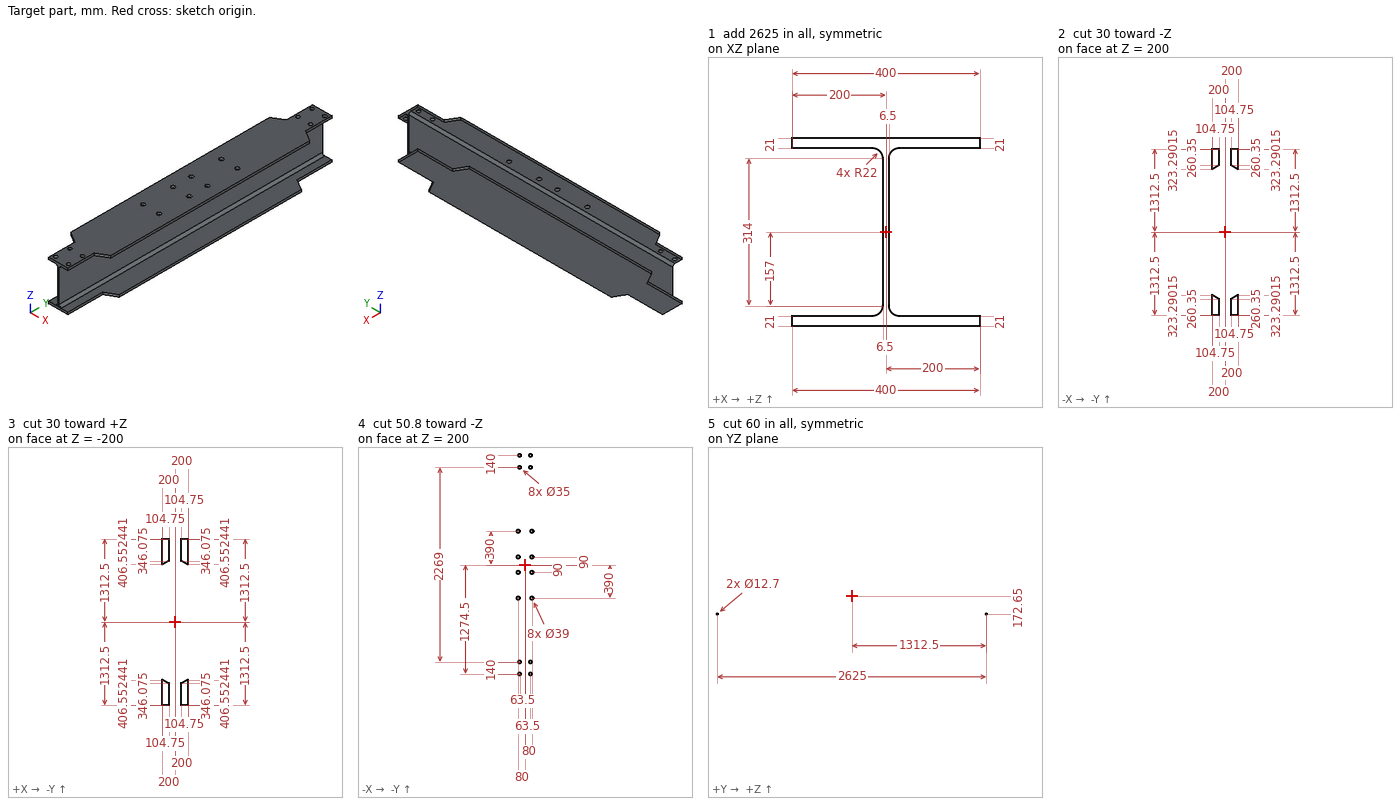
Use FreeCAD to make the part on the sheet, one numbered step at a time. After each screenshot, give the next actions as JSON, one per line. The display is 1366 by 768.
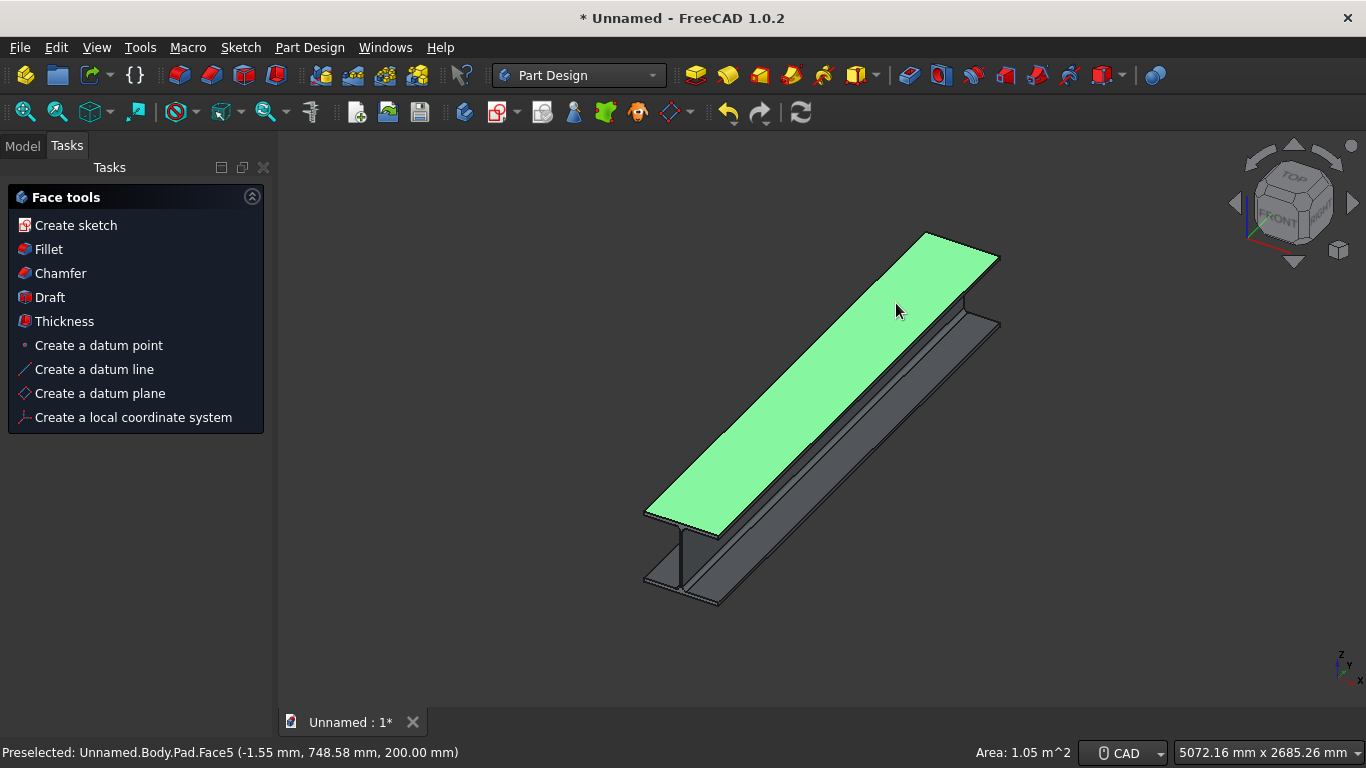
{"action": "left_click", "coordinate": [498, 112]}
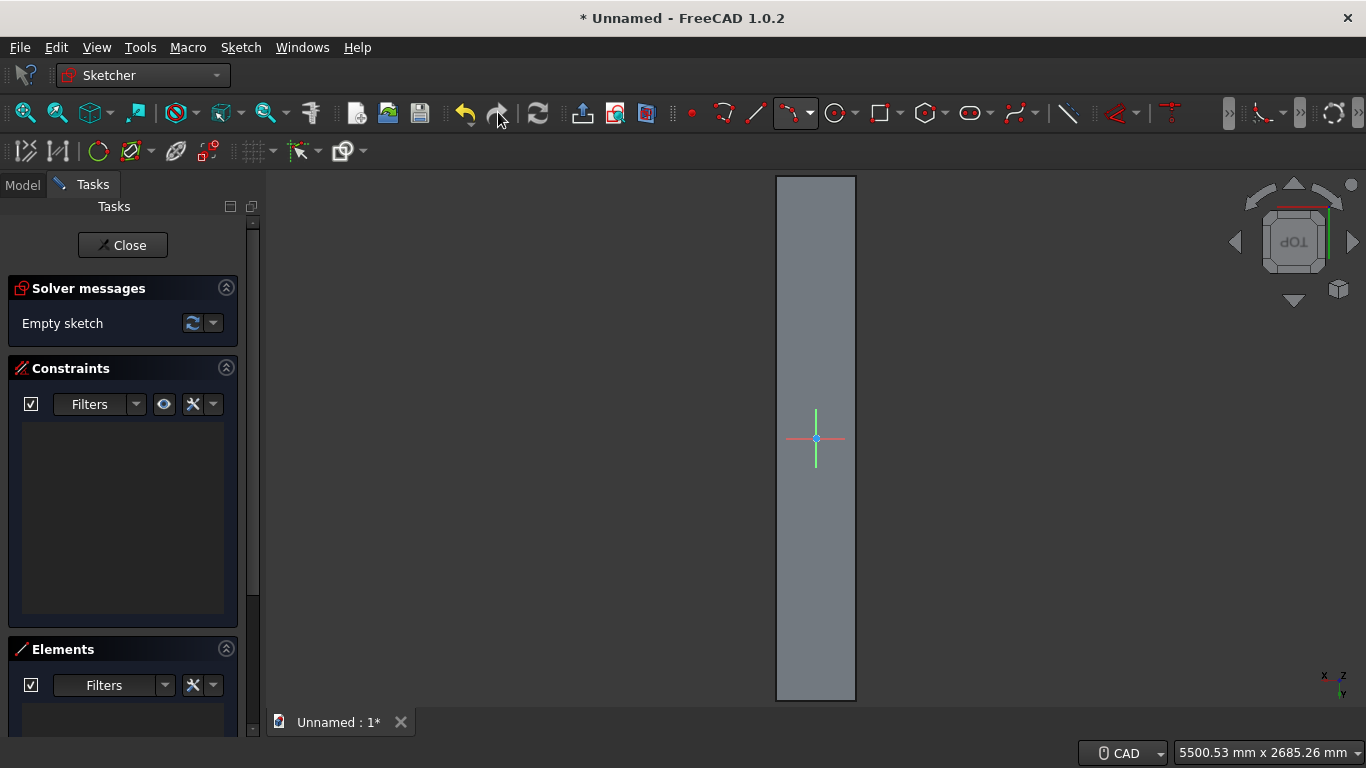
{"action": "scroll", "coordinate": [608, 438], "scroll_direction": "down", "scroll_amount": 2}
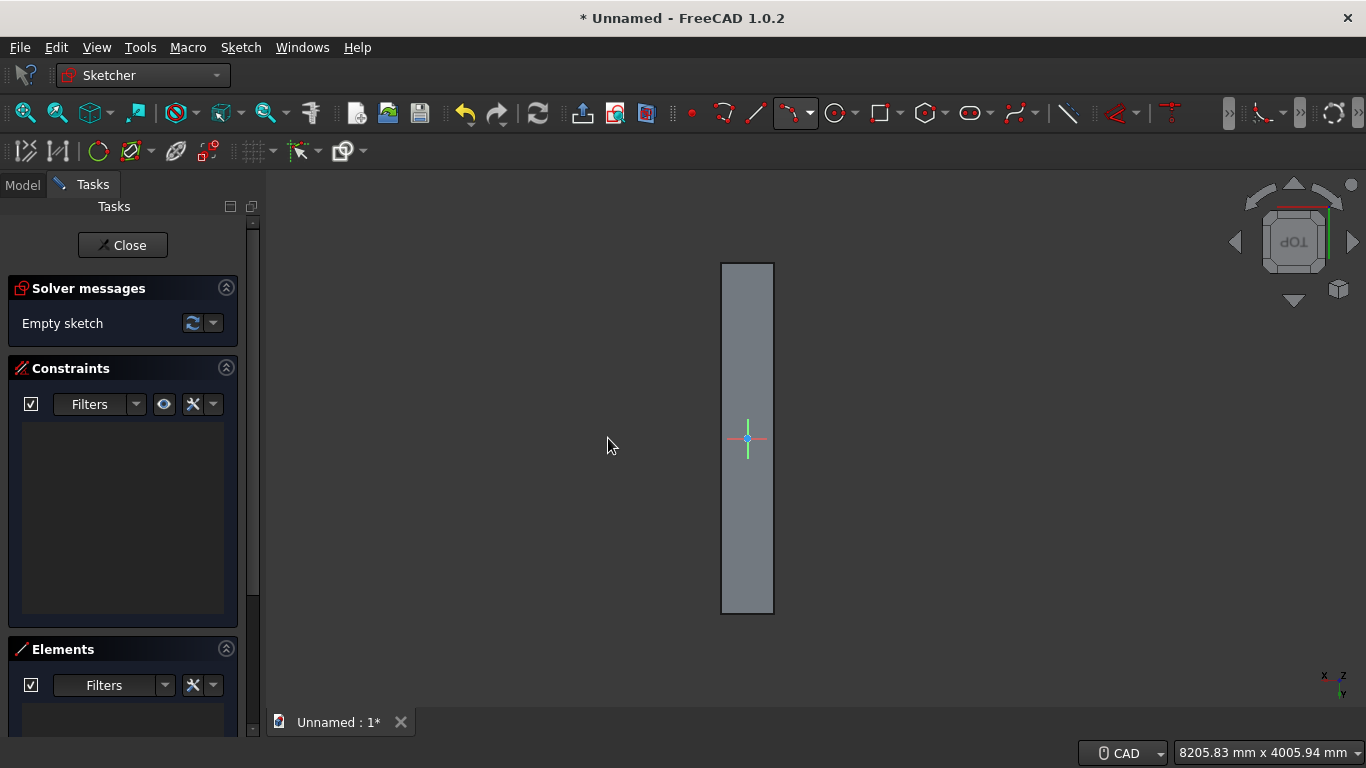
{"action": "left_click", "coordinate": [724, 114]}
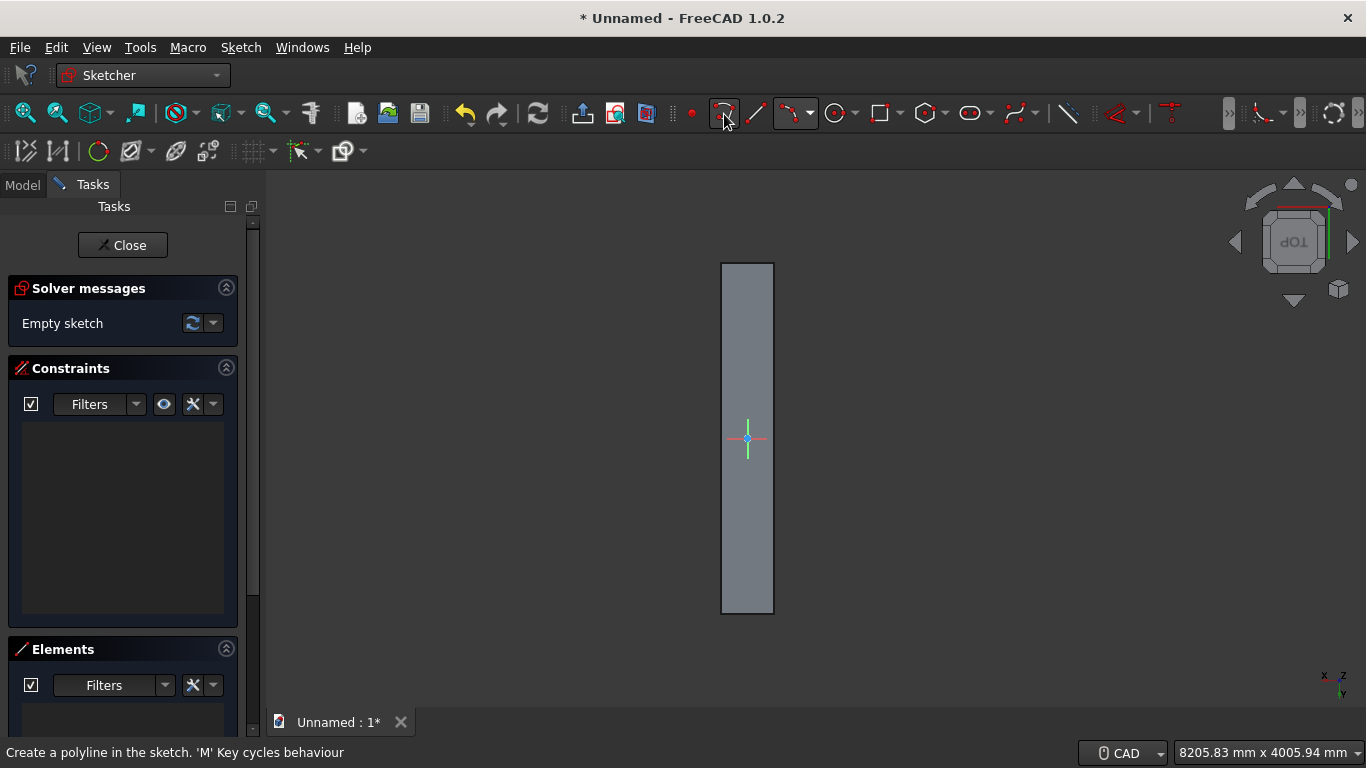
{"action": "left_click", "coordinate": [774, 571]}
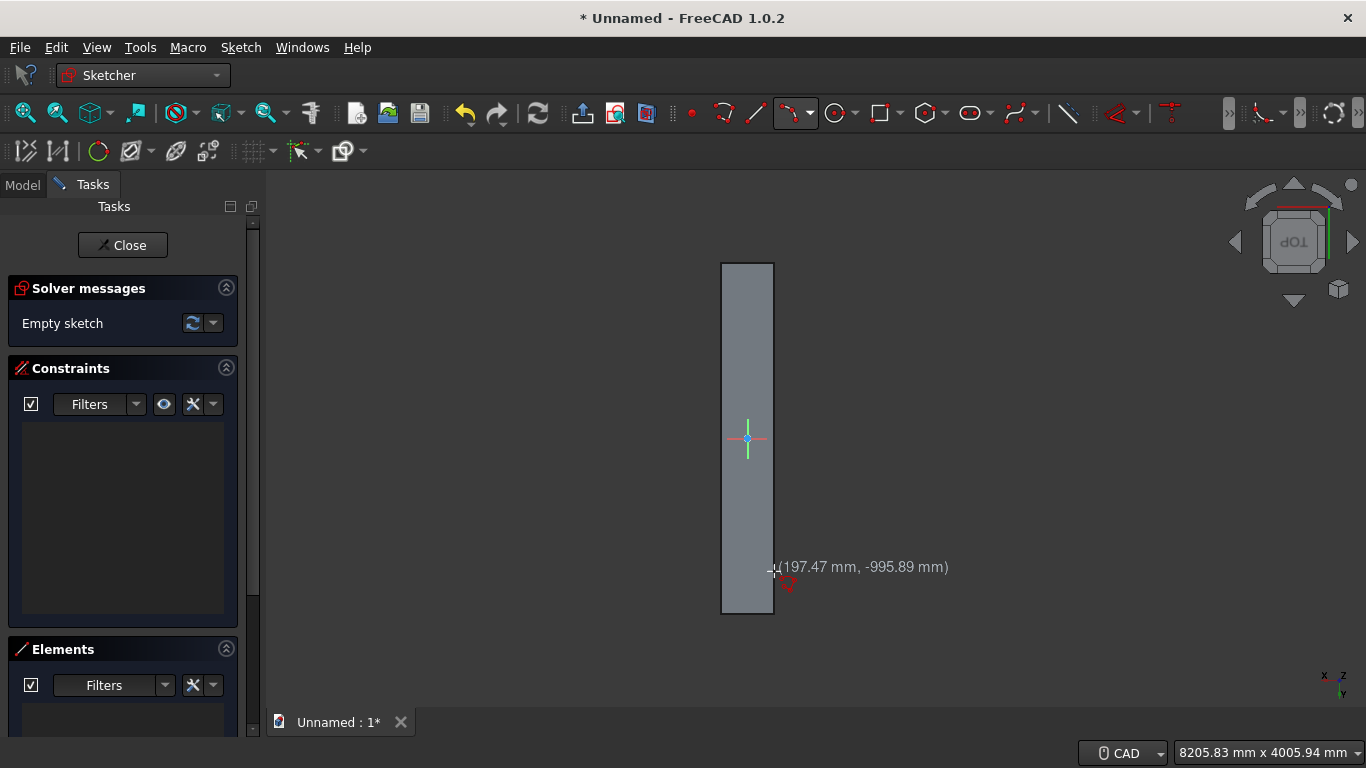
{"action": "scroll", "coordinate": [760, 580], "scroll_direction": "up", "scroll_amount": 2}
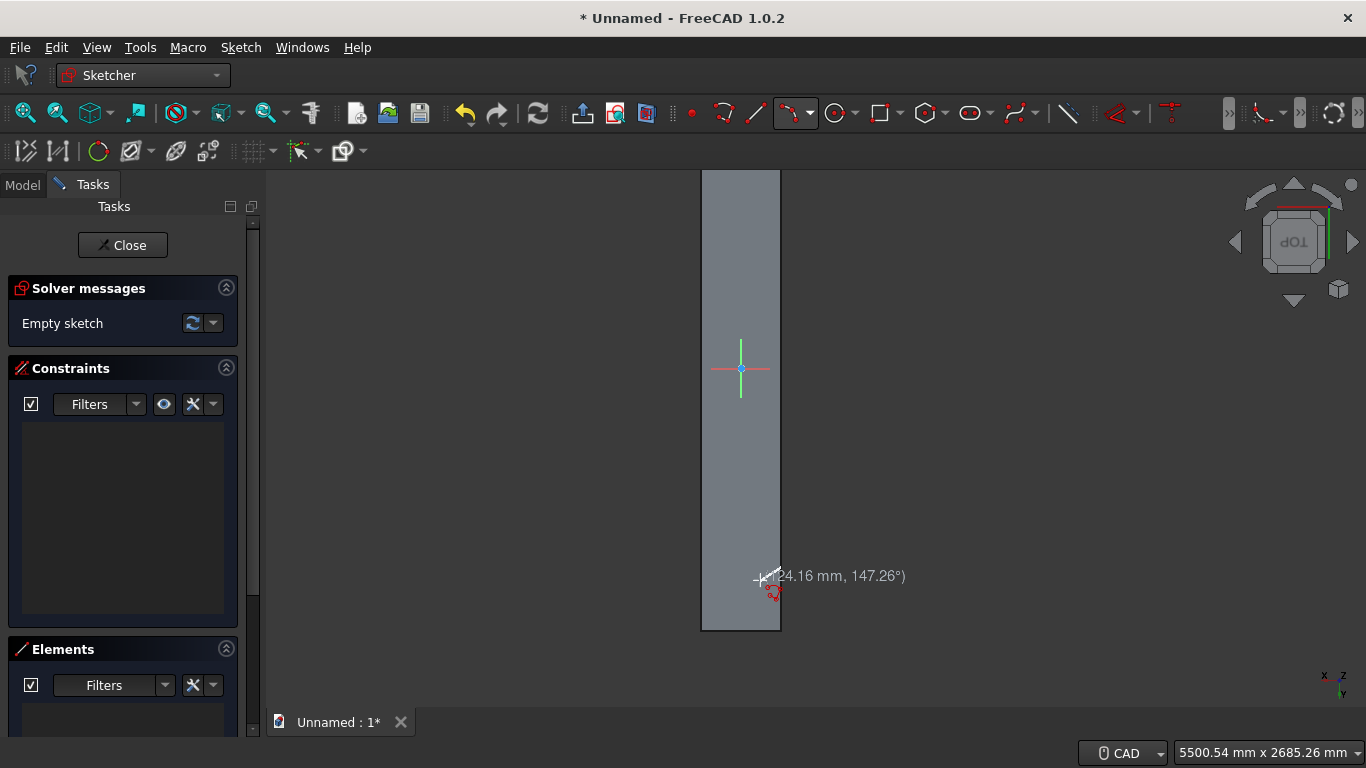
{"action": "left_click", "coordinate": [760, 579]}
{"action": "left_click", "coordinate": [760, 631]}
{"action": "left_click", "coordinate": [781, 631]}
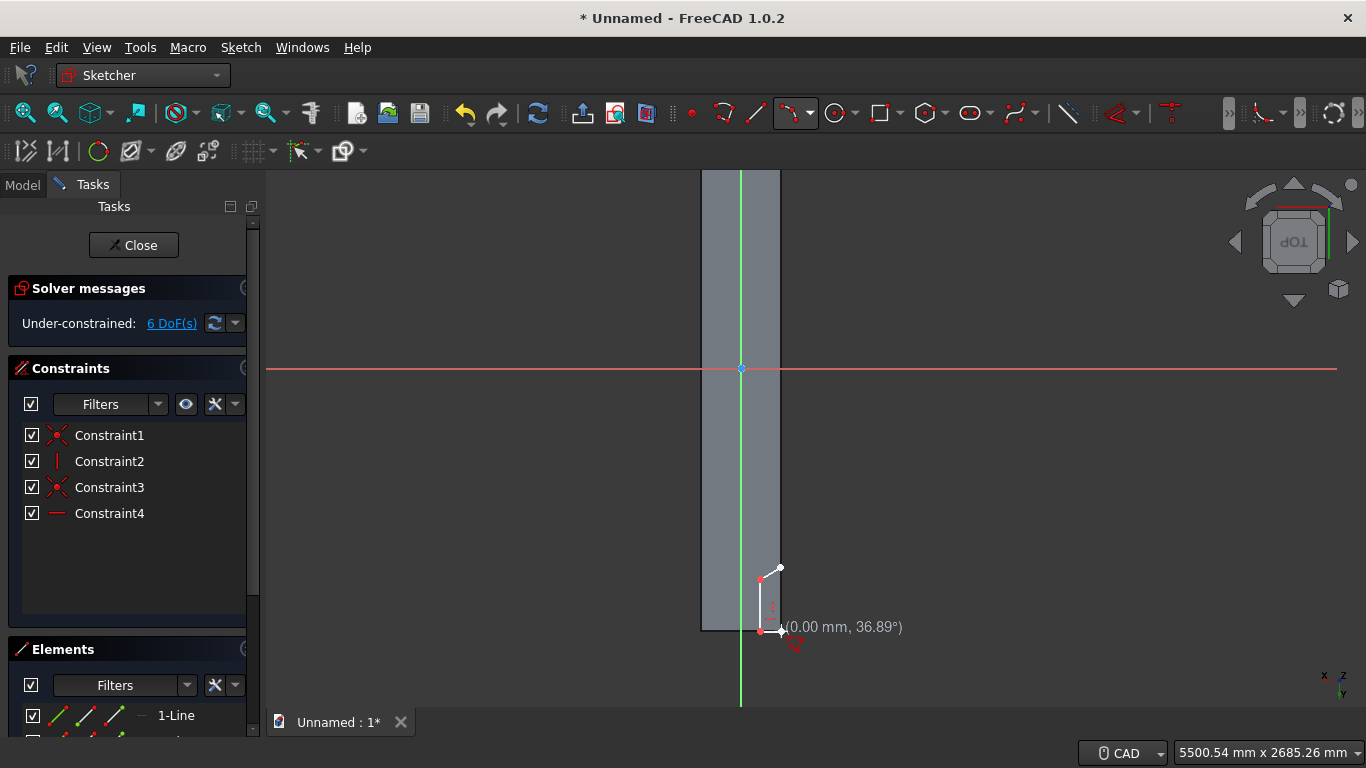
{"action": "scroll", "coordinate": [781, 566], "scroll_direction": "up", "scroll_amount": 2}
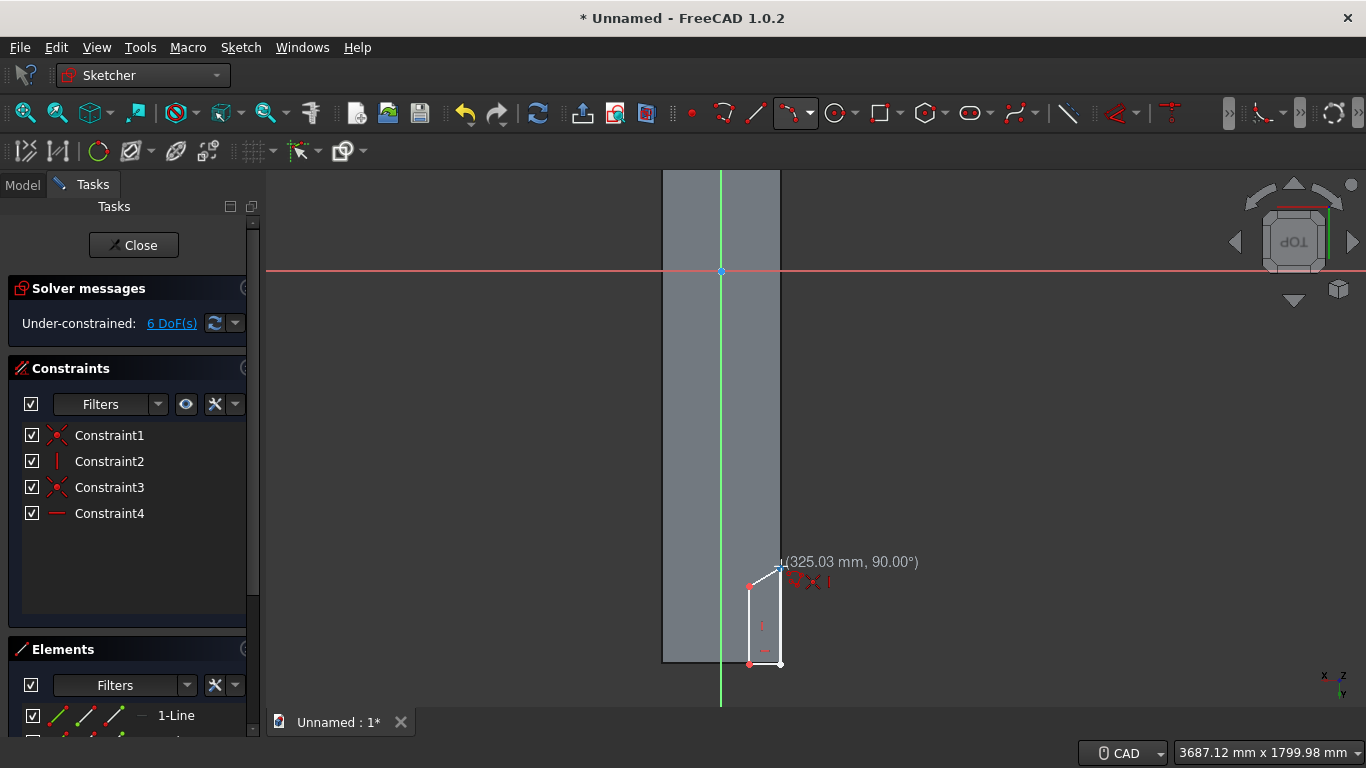
{"action": "left_click", "coordinate": [780, 568]}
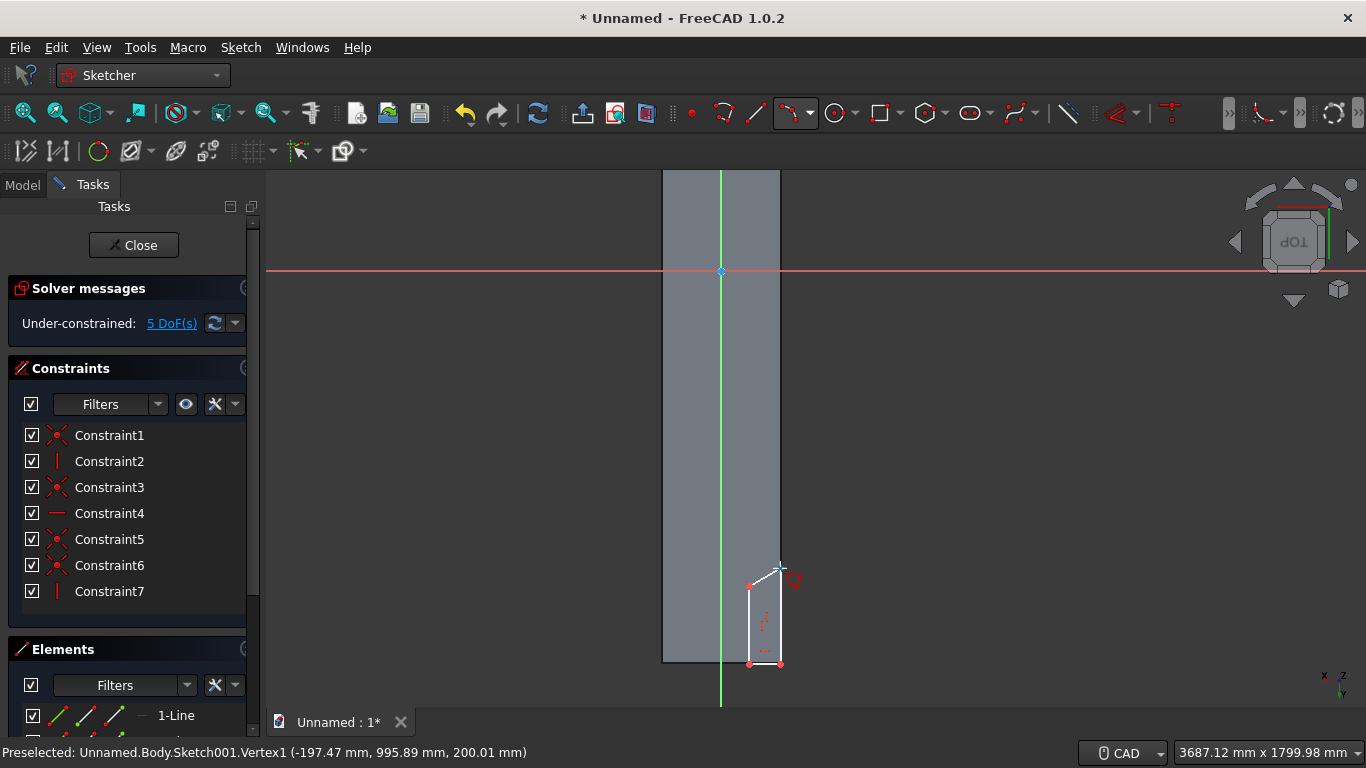
{"action": "left_click", "coordinate": [662, 566]}
{"action": "left_click", "coordinate": [662, 663]}
{"action": "left_click", "coordinate": [693, 663]}
{"action": "left_click", "coordinate": [693, 585]}
{"action": "left_click", "coordinate": [662, 567]}